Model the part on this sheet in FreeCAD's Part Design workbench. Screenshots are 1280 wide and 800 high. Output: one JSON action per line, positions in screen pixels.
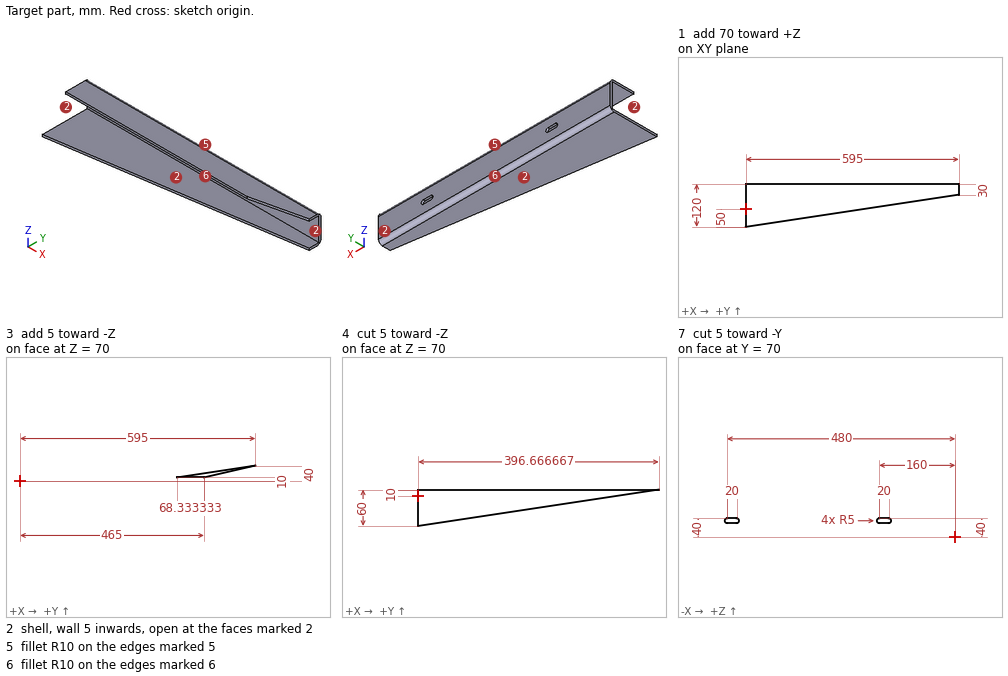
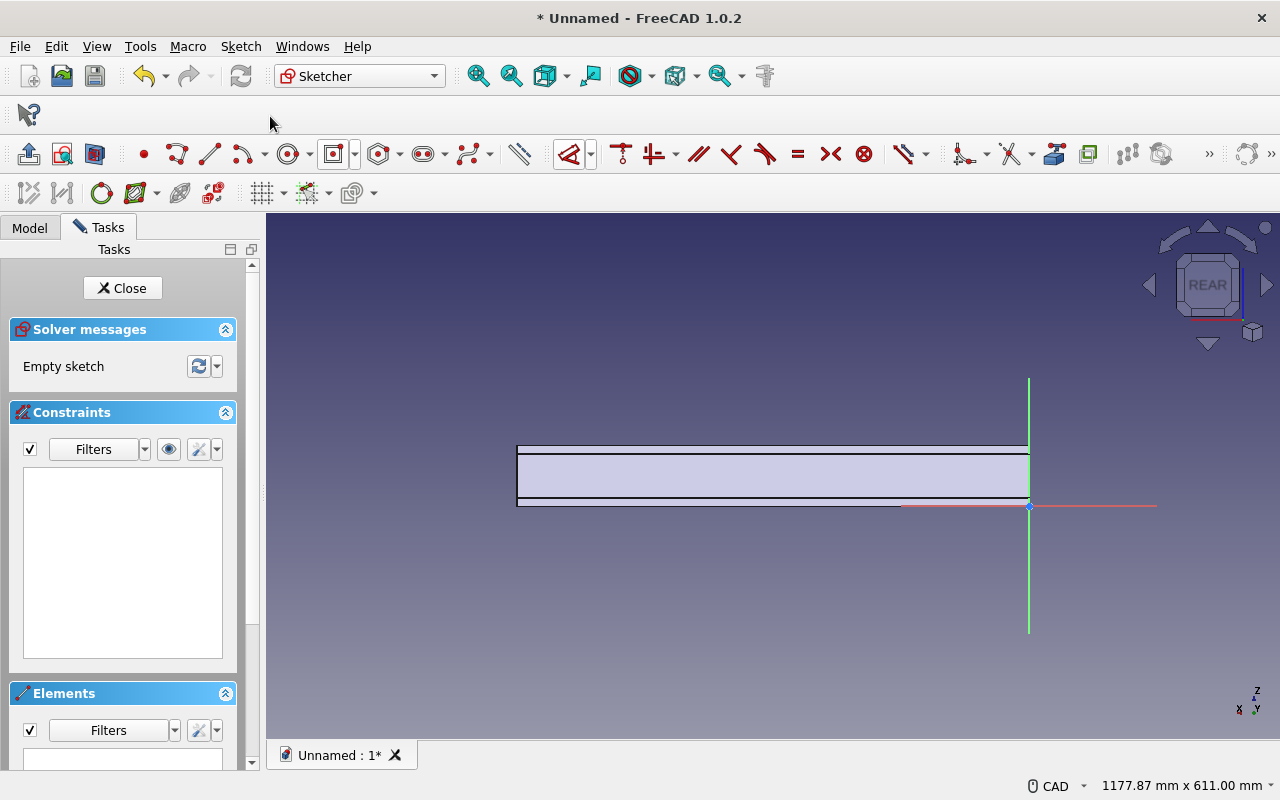
{"action": "scroll", "coordinate": [1056, 515], "scroll_direction": "up", "scroll_amount": 2}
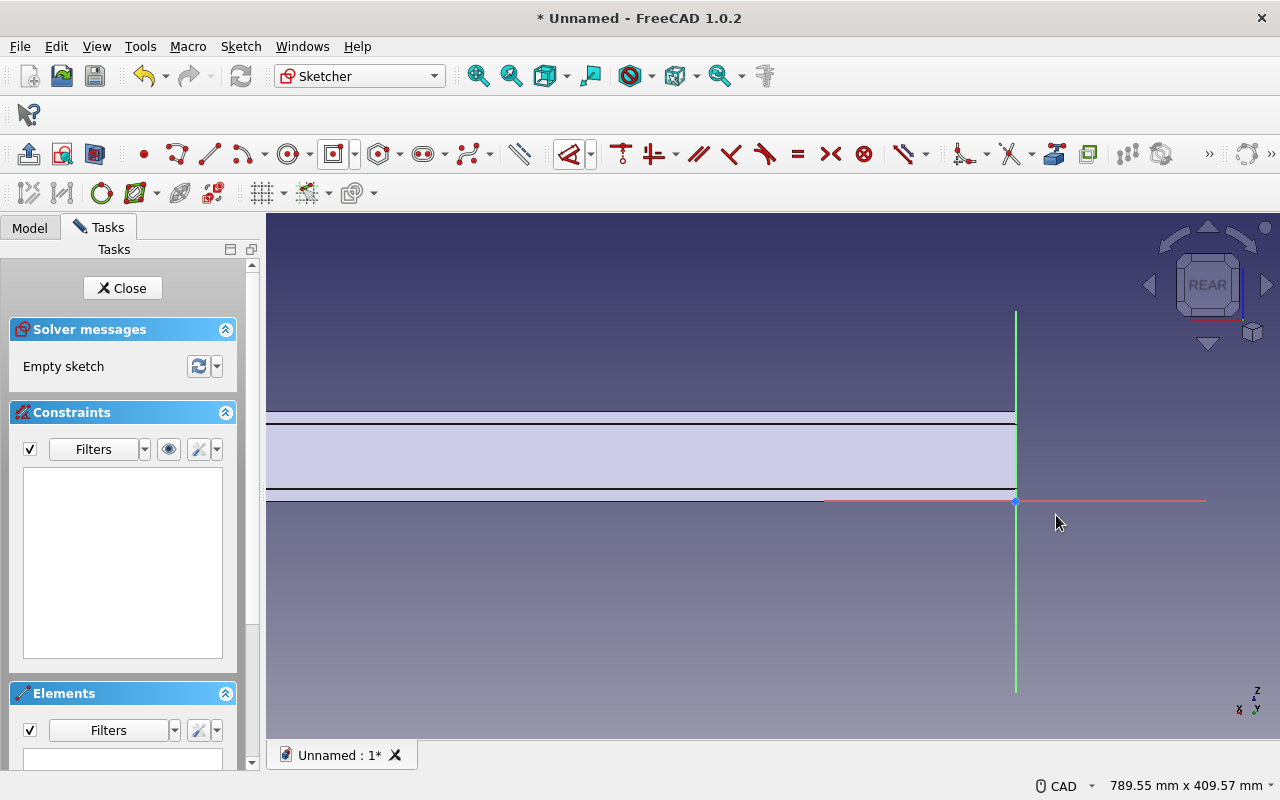
{"action": "left_click", "coordinate": [422, 154]}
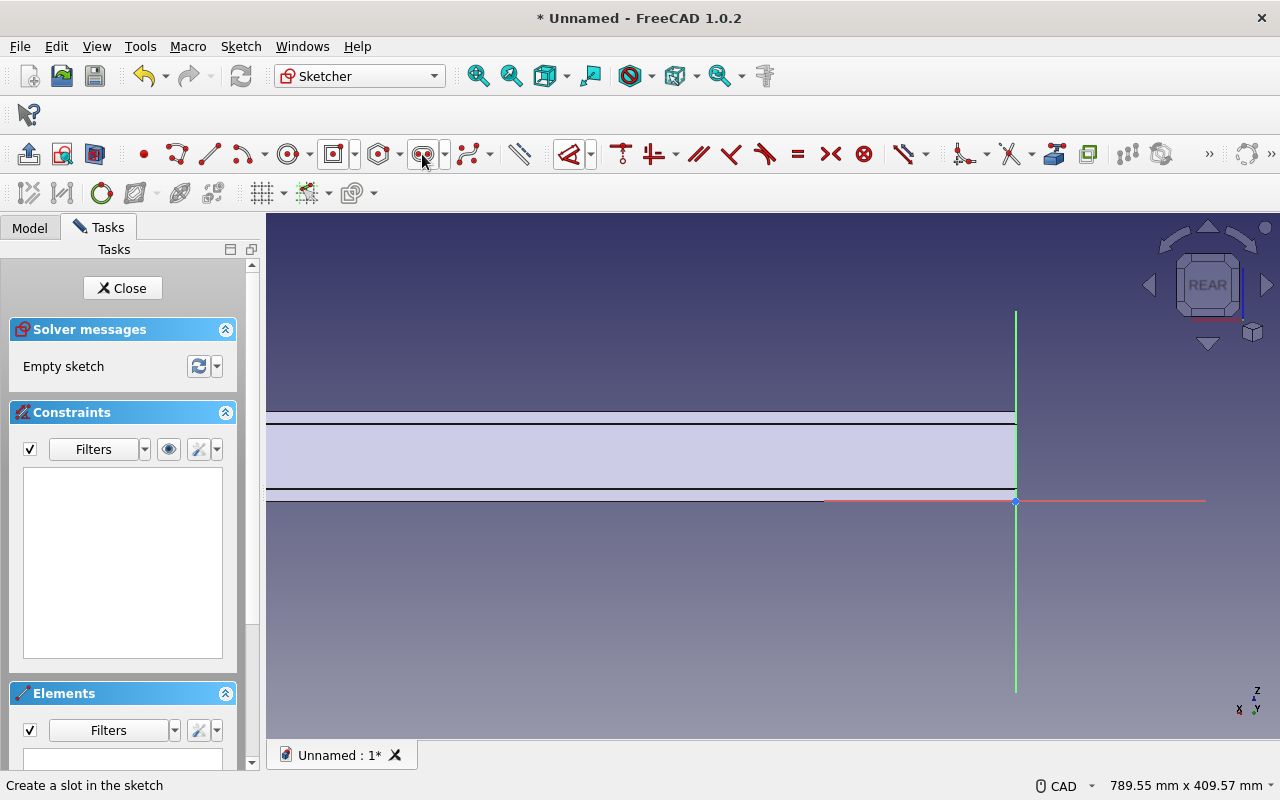
{"action": "scroll", "coordinate": [810, 457], "scroll_direction": "up", "scroll_amount": 7}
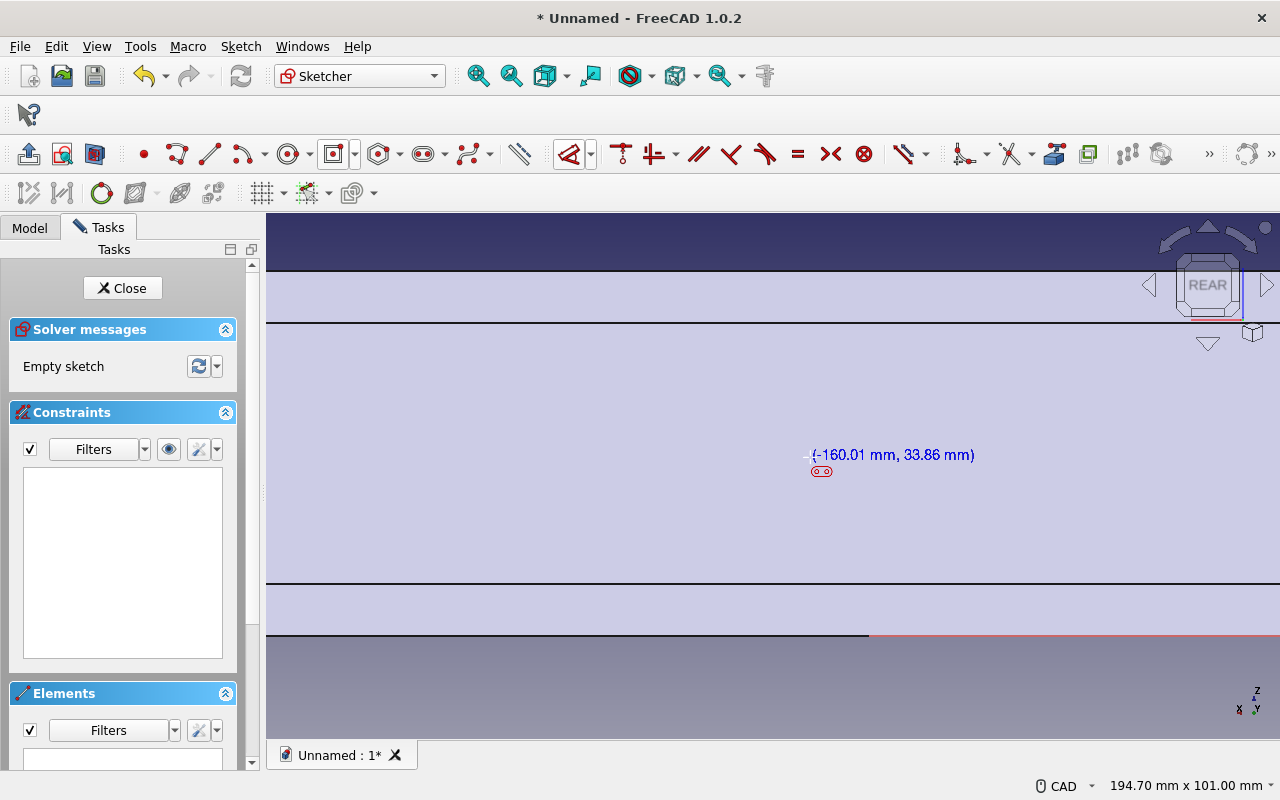
{"action": "scroll", "coordinate": [811, 458], "scroll_direction": "down", "scroll_amount": 7}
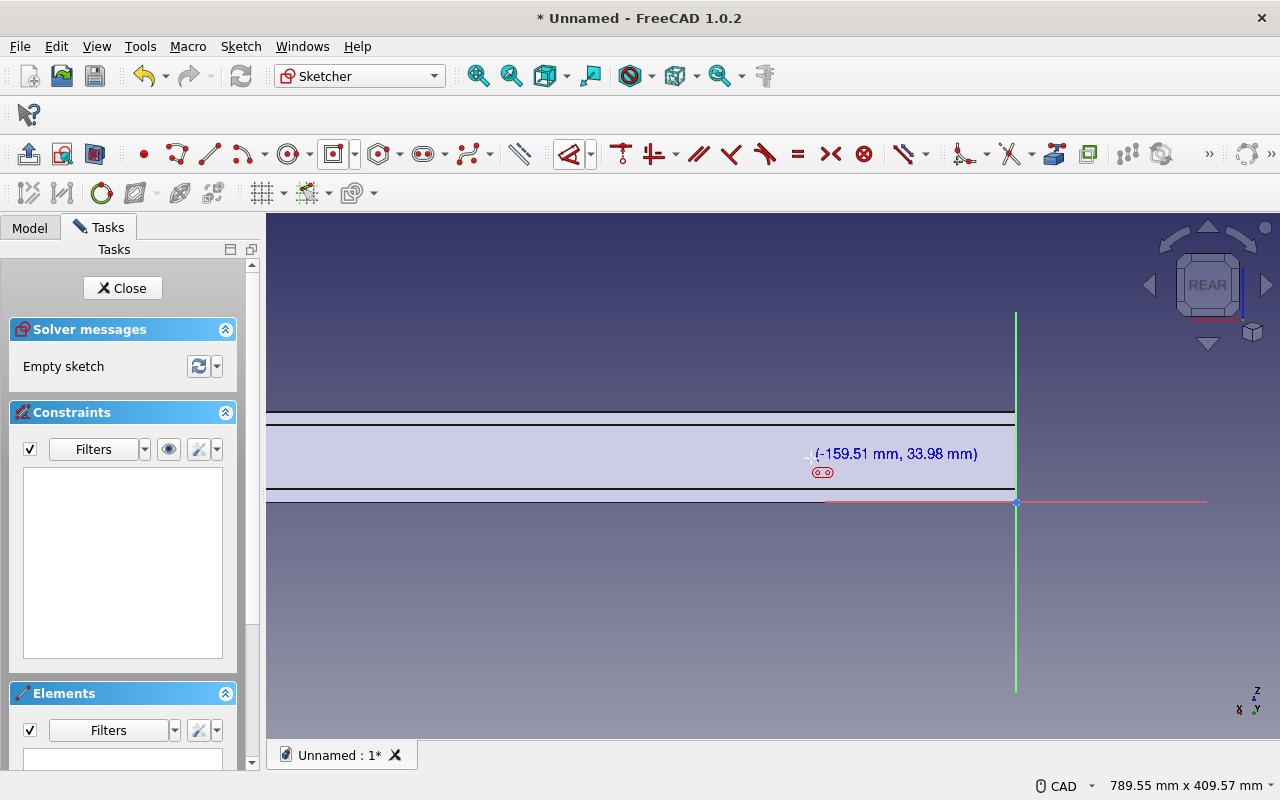
{"action": "left_click", "coordinate": [811, 457]}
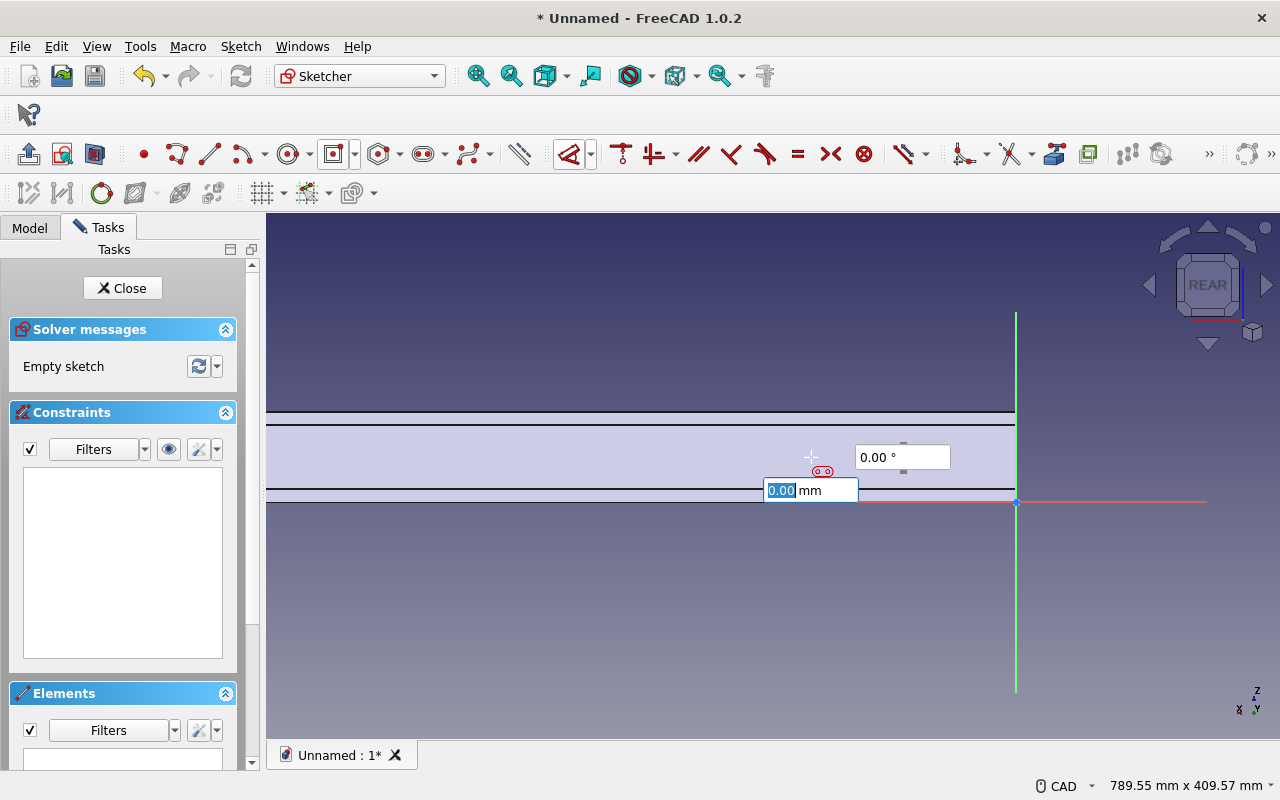
{"action": "left_click", "coordinate": [836, 457]}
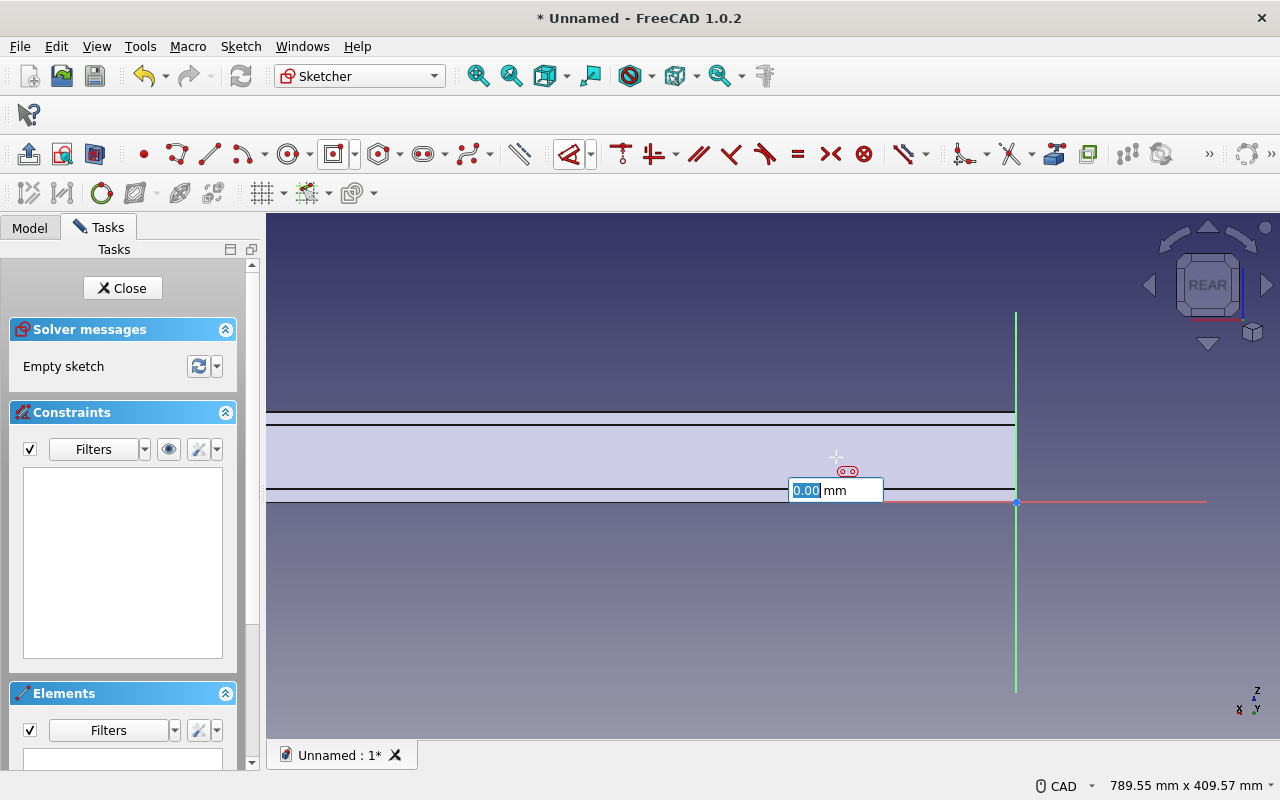
{"action": "scroll", "coordinate": [824, 451], "scroll_direction": "up", "scroll_amount": 5}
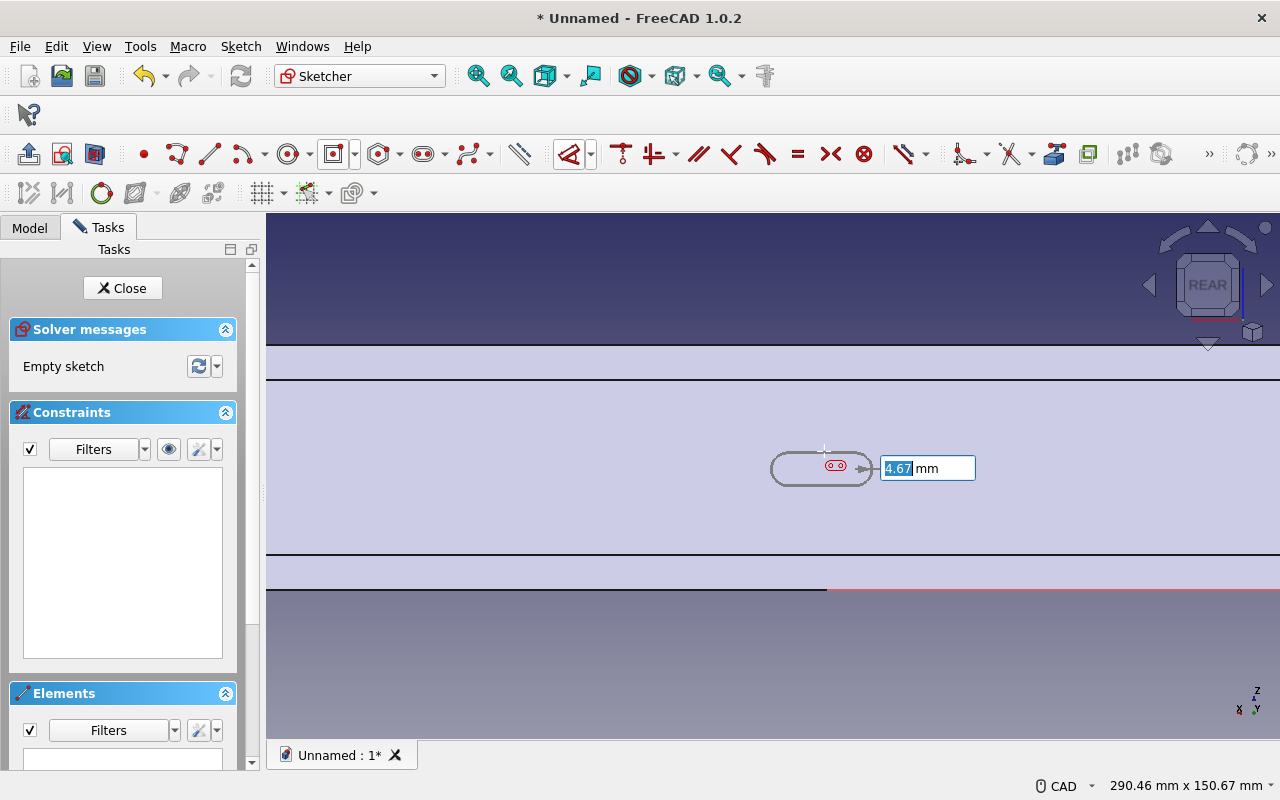
{"action": "left_click", "coordinate": [822, 450]}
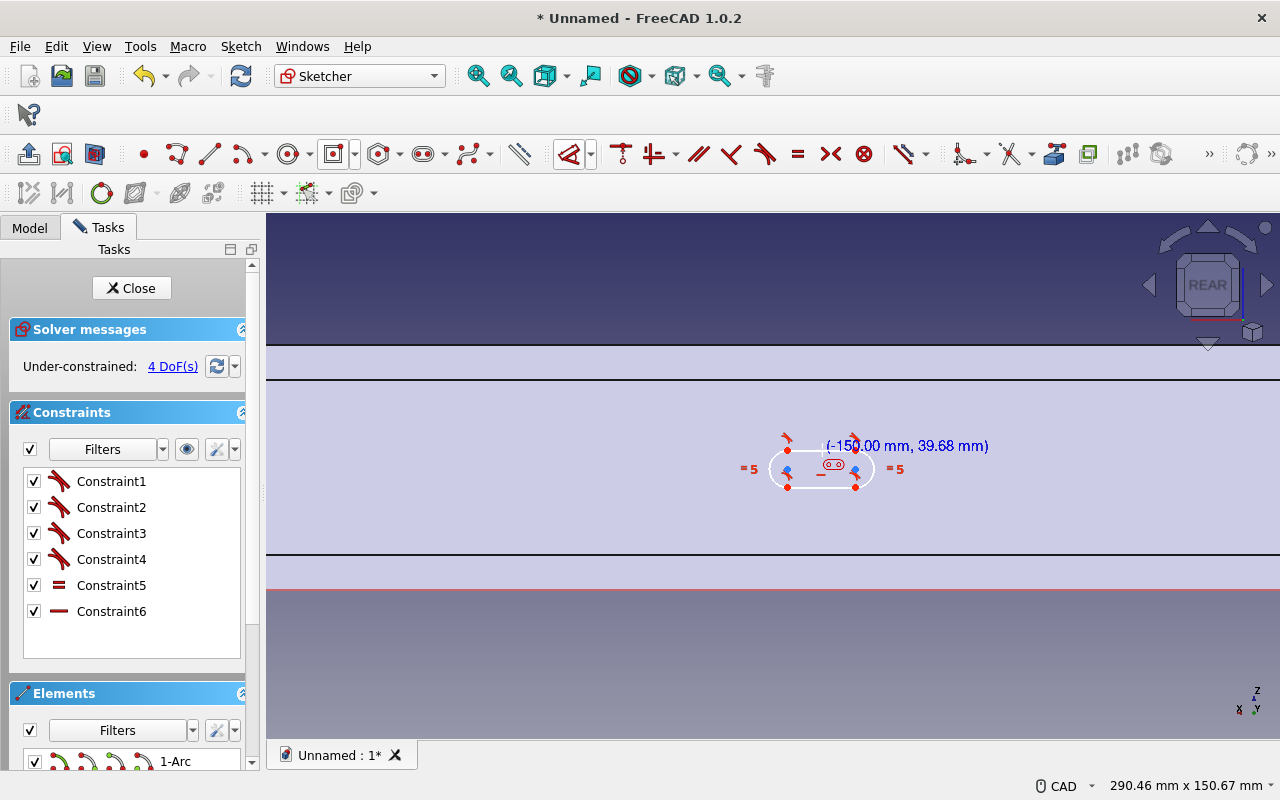
{"action": "scroll", "coordinate": [824, 451], "scroll_direction": "down", "scroll_amount": 5}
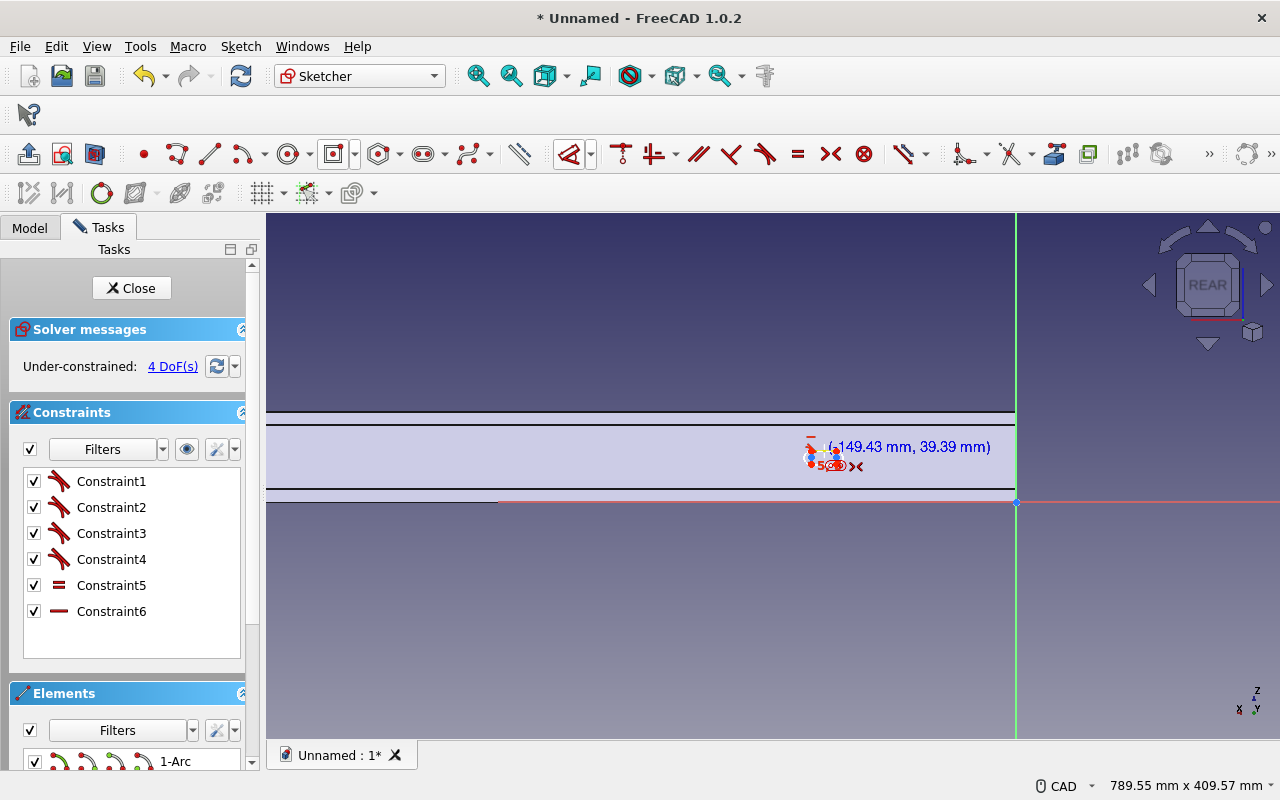
{"action": "scroll", "coordinate": [400, 457], "scroll_direction": "up", "scroll_amount": 7}